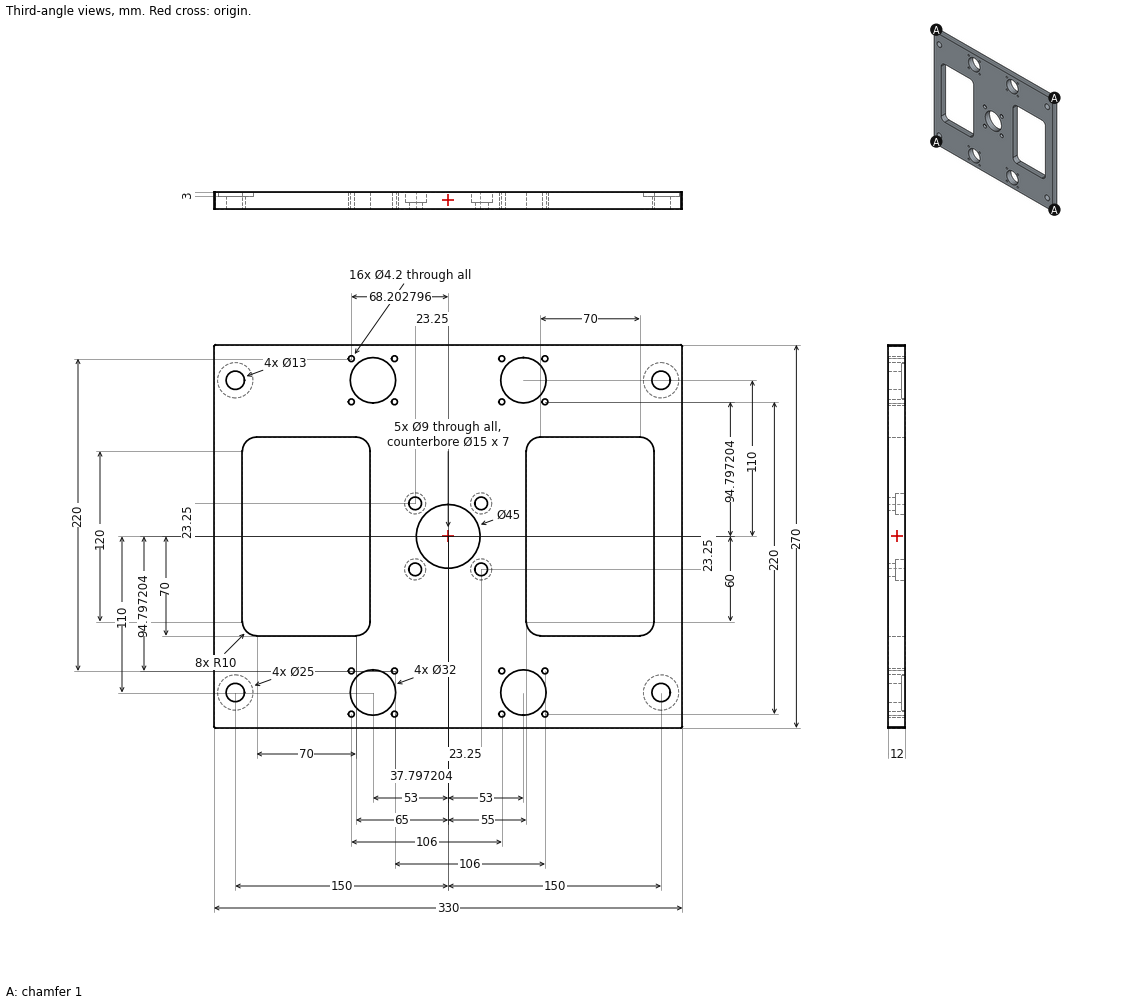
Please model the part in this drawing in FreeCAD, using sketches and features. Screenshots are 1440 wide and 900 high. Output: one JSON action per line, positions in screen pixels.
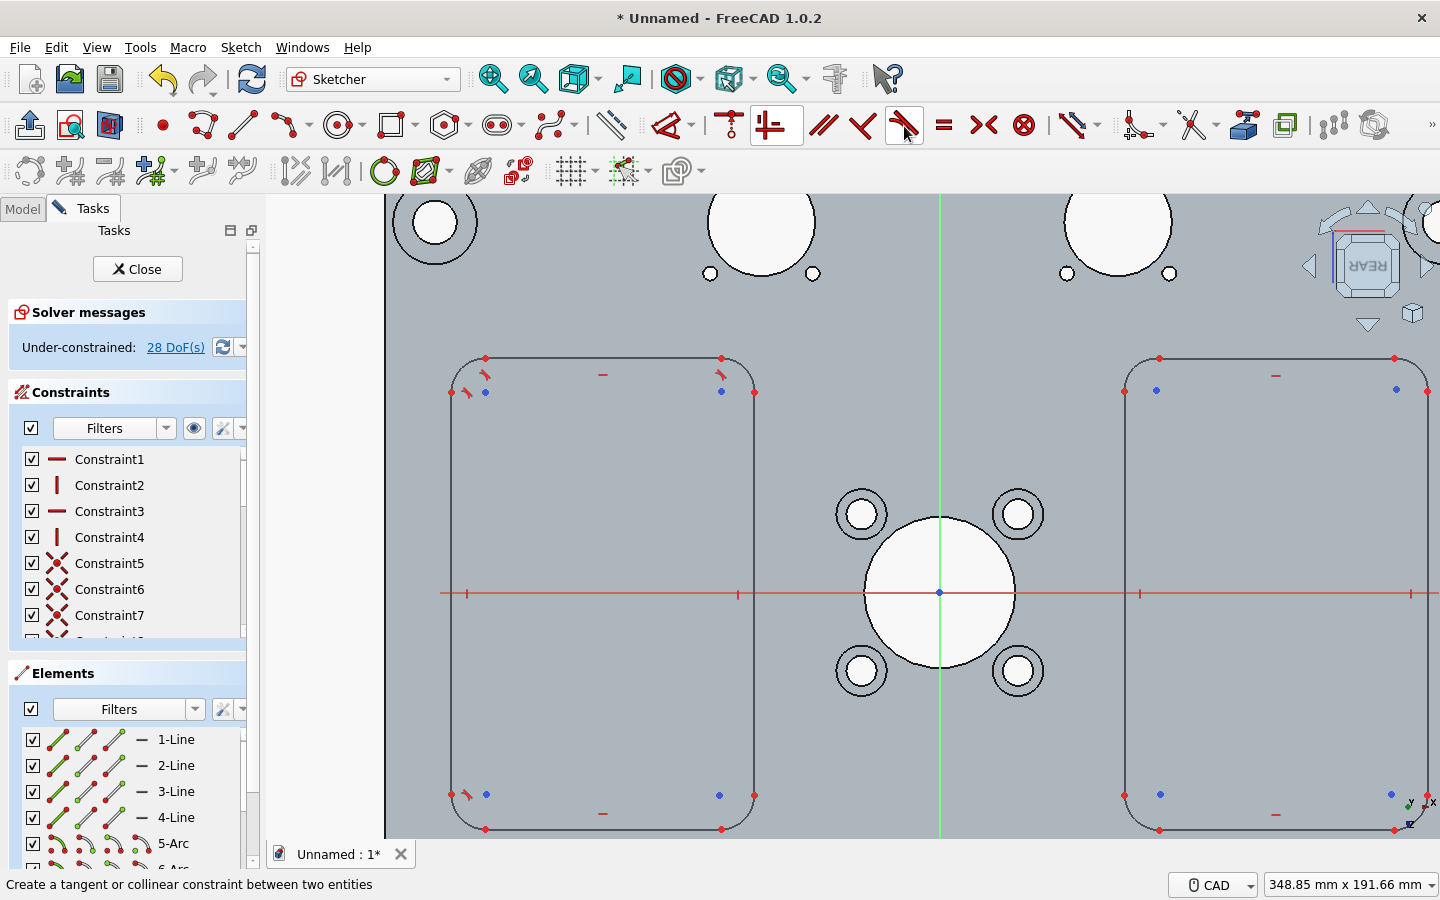
{"action": "scroll", "coordinate": [469, 362], "scroll_direction": "down", "scroll_amount": 2}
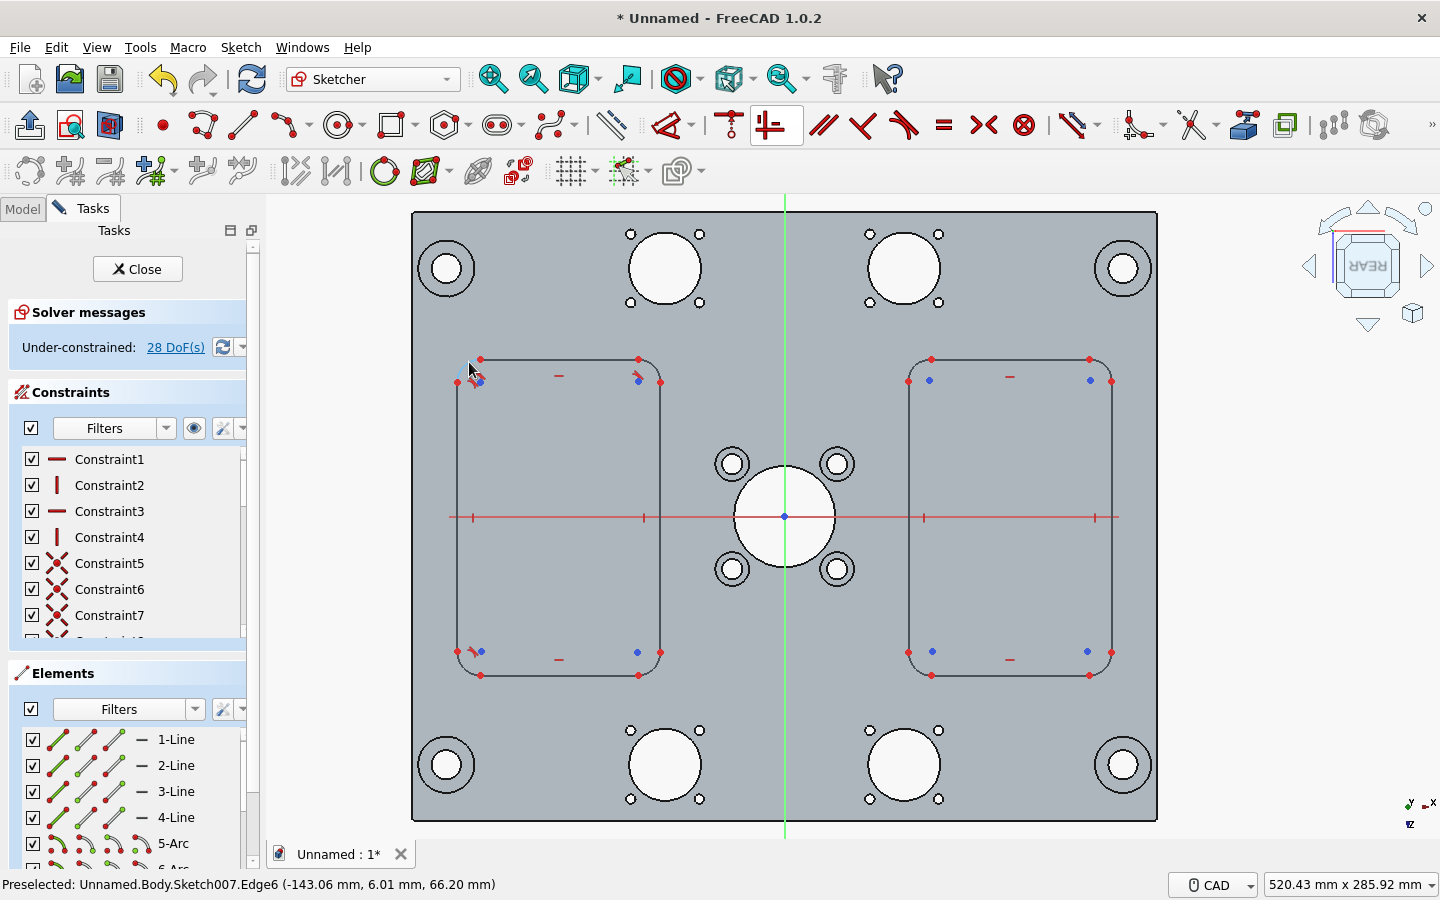
{"action": "left_click", "coordinate": [528, 676]}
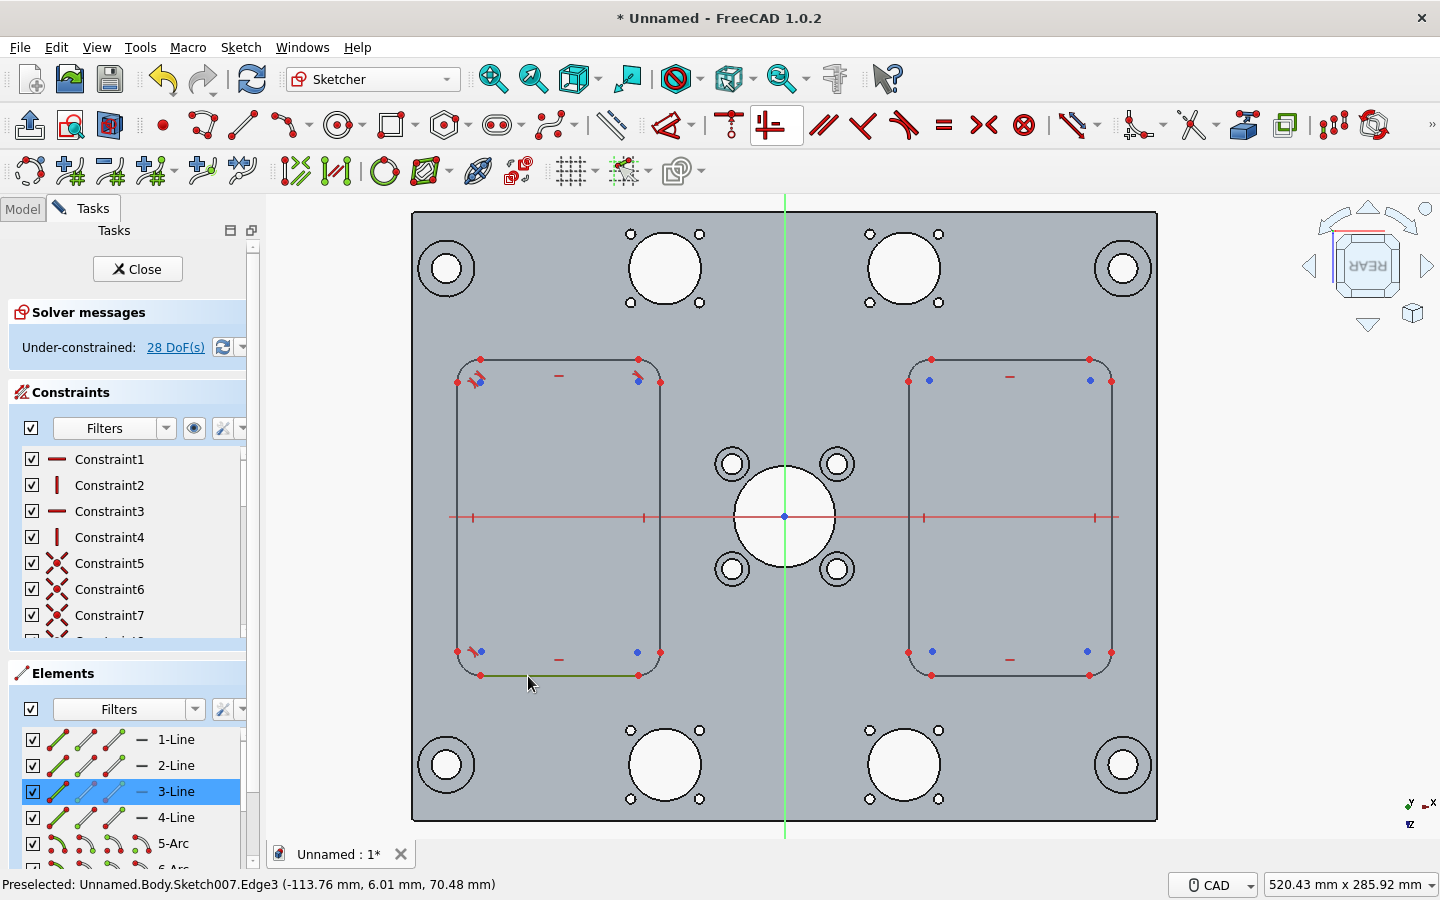
{"action": "scroll", "coordinate": [460, 662], "scroll_direction": "up", "scroll_amount": 2}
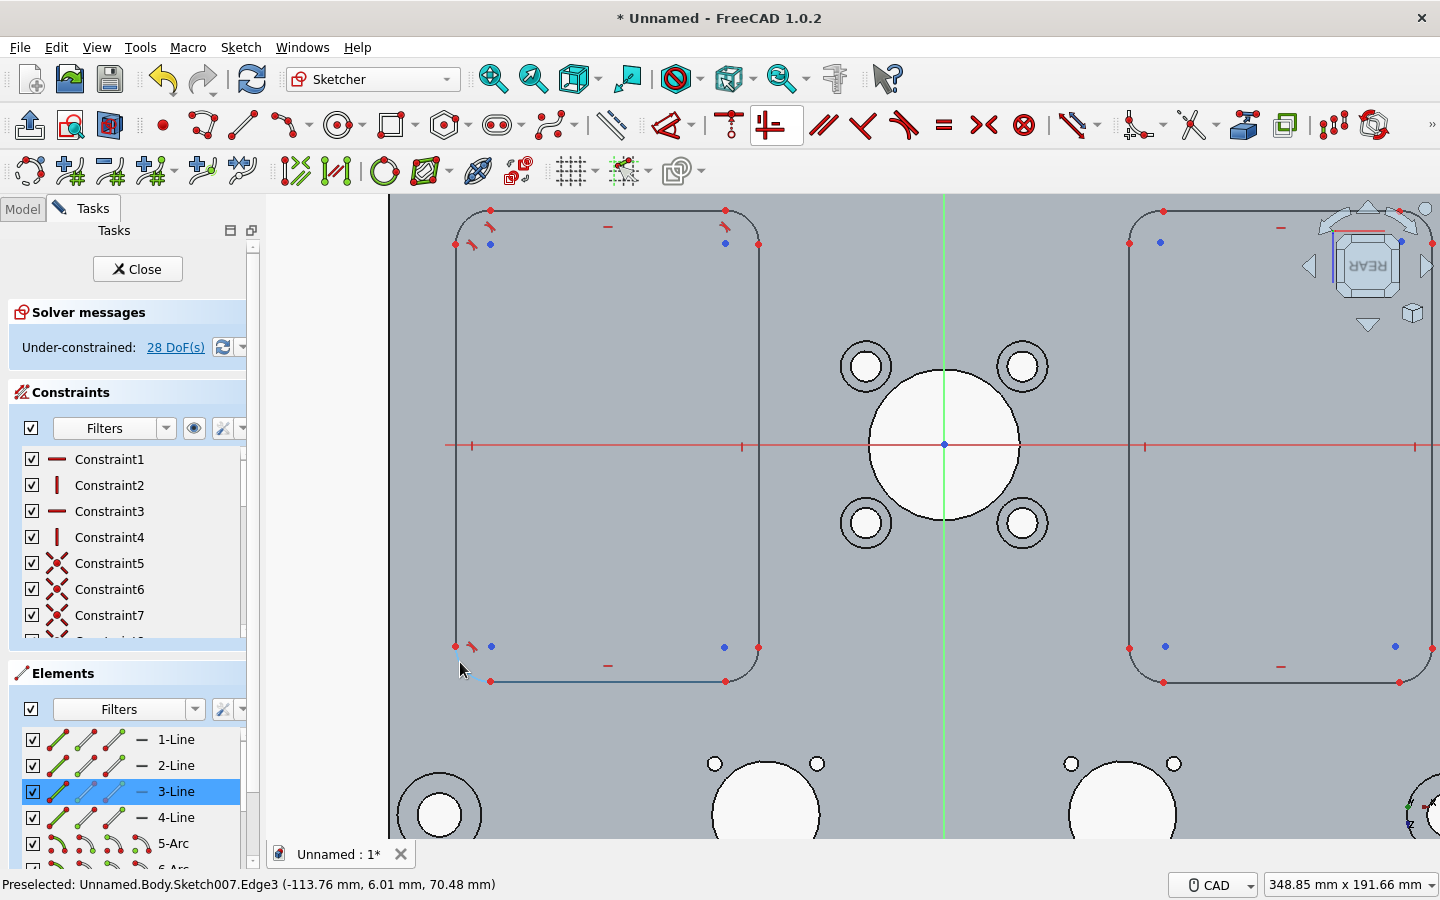
{"action": "left_click", "coordinate": [460, 662]}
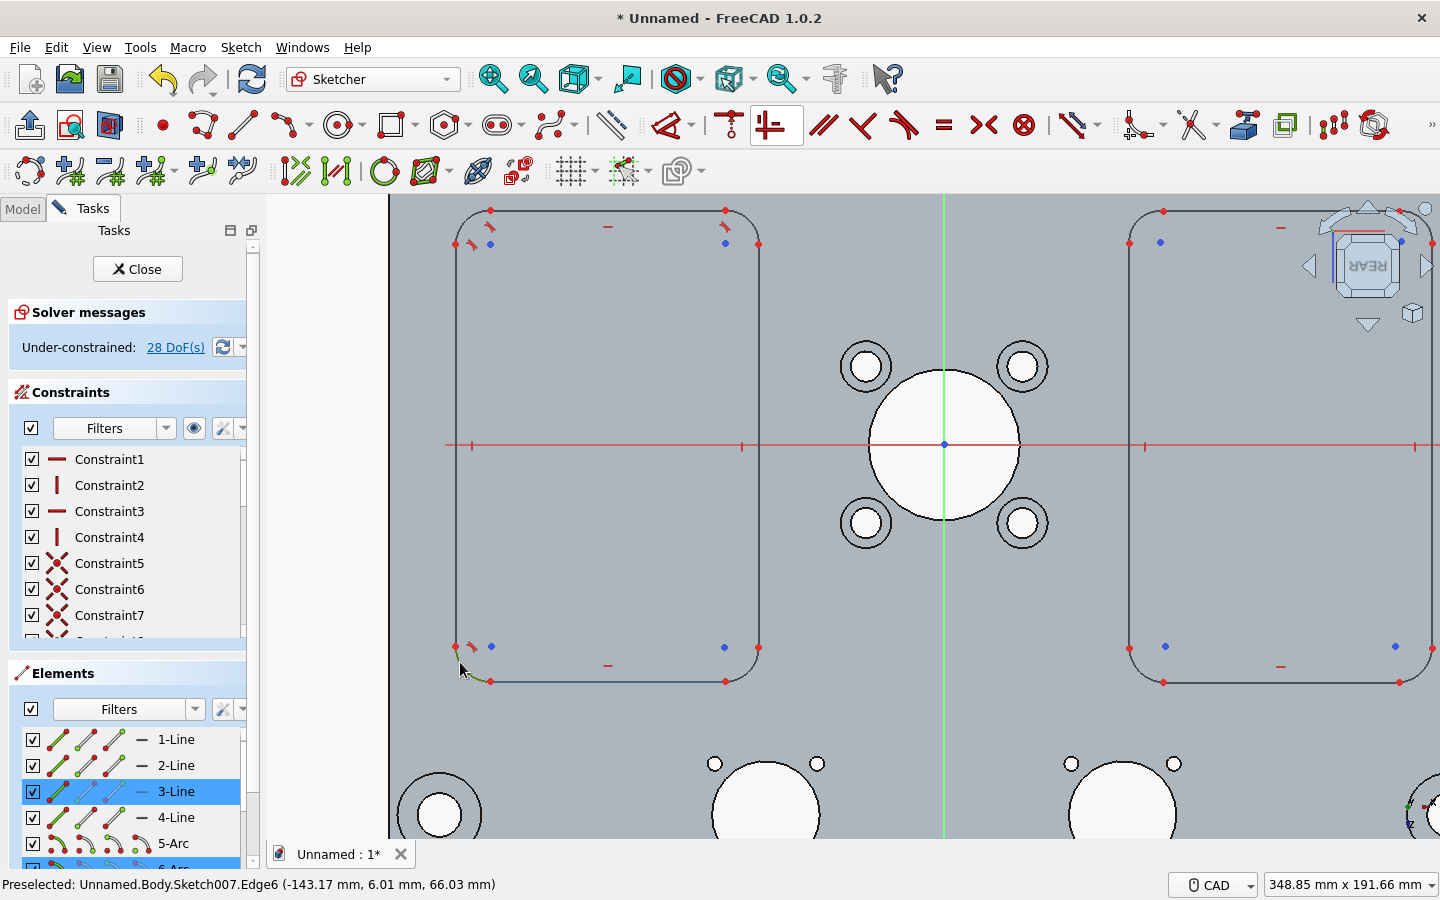
{"action": "left_click", "coordinate": [904, 126]}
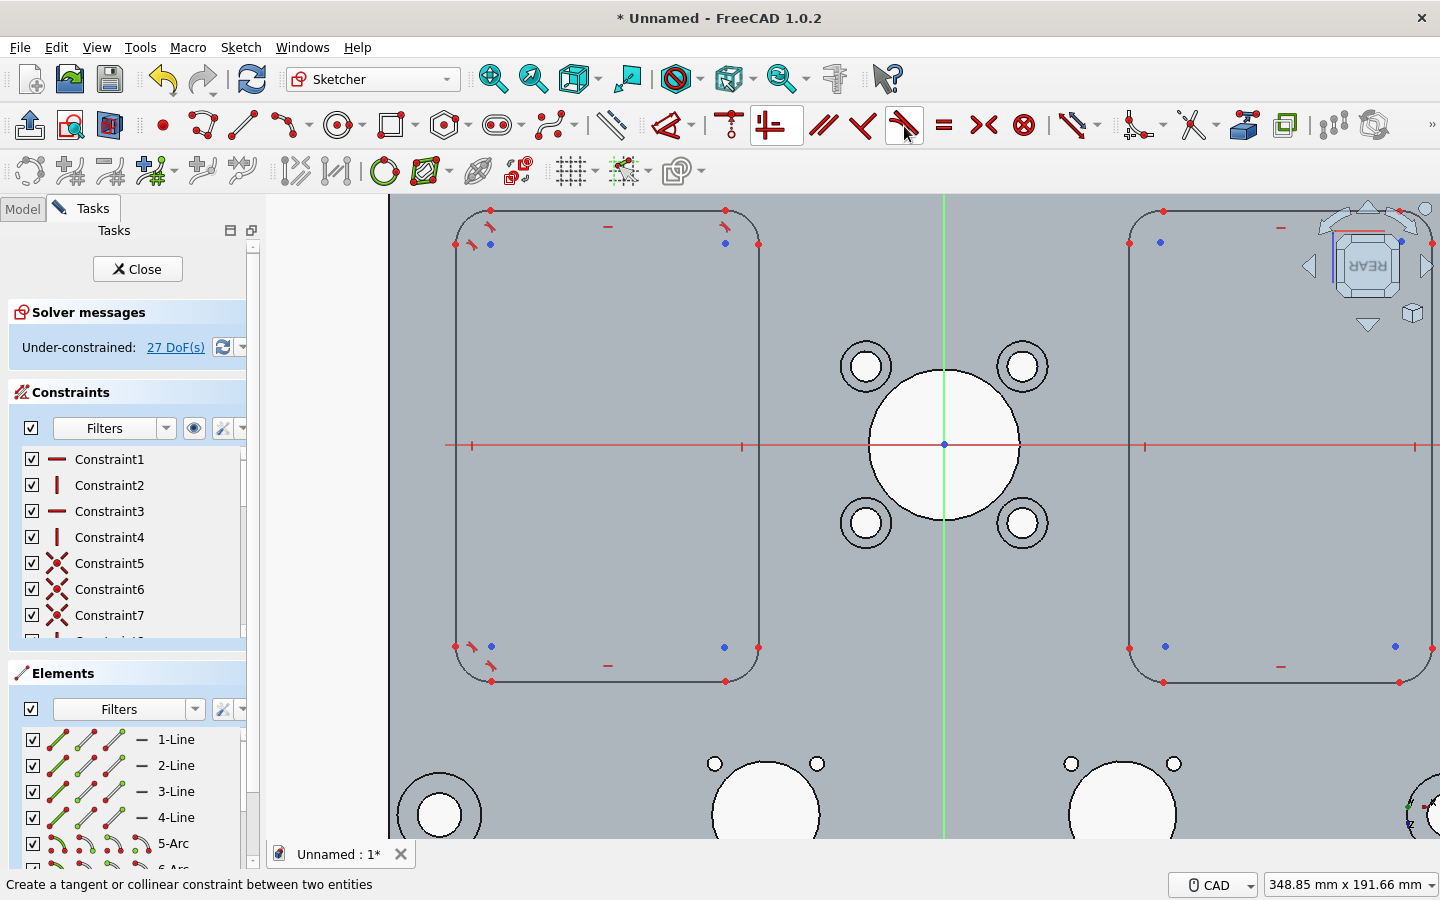
{"action": "left_click", "coordinate": [562, 682]}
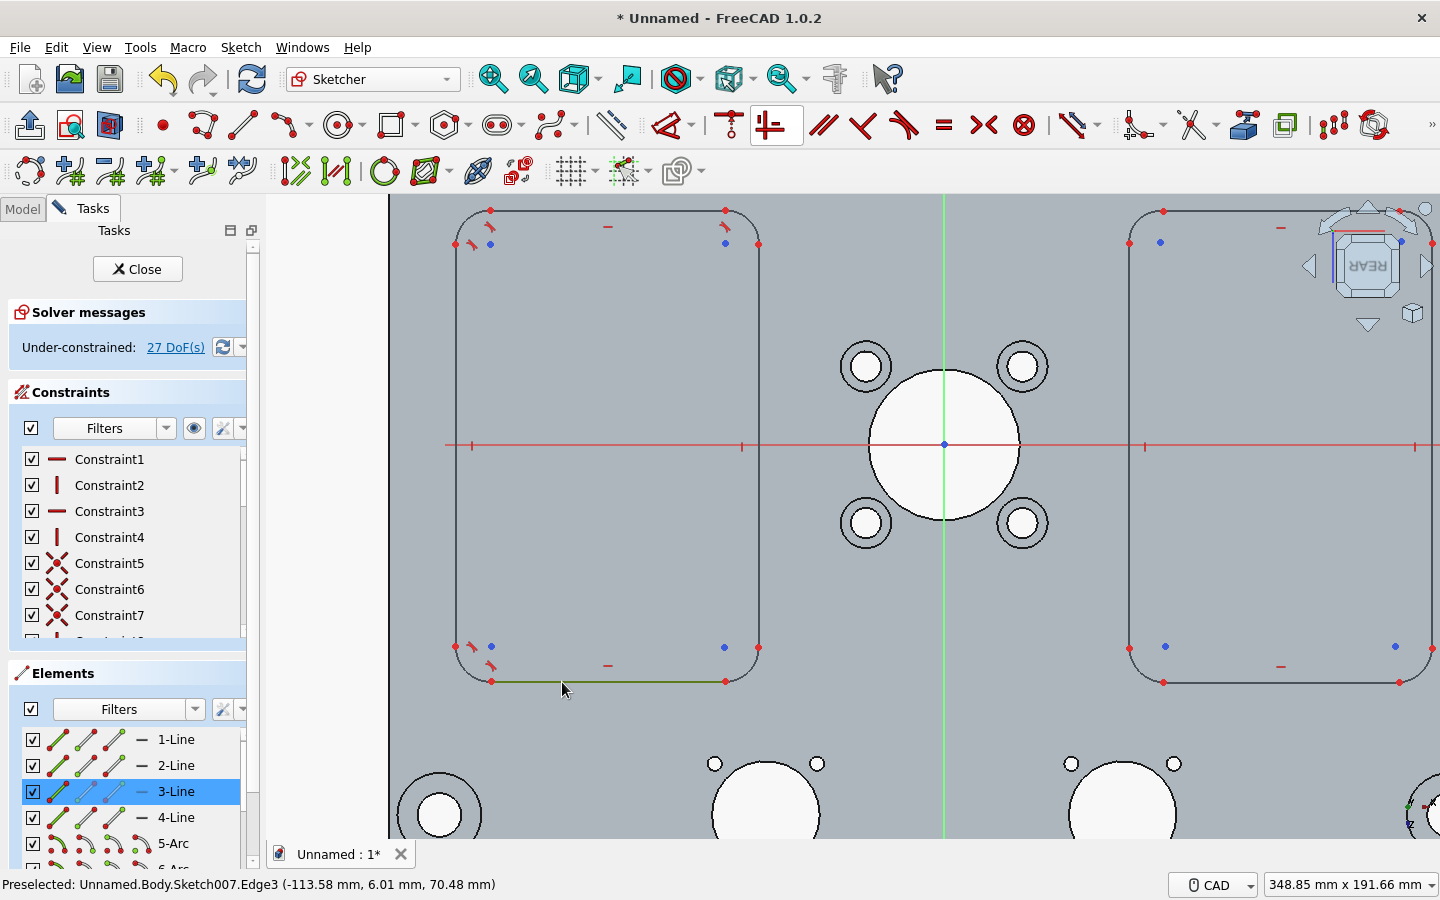
{"action": "left_click", "coordinate": [741, 678]}